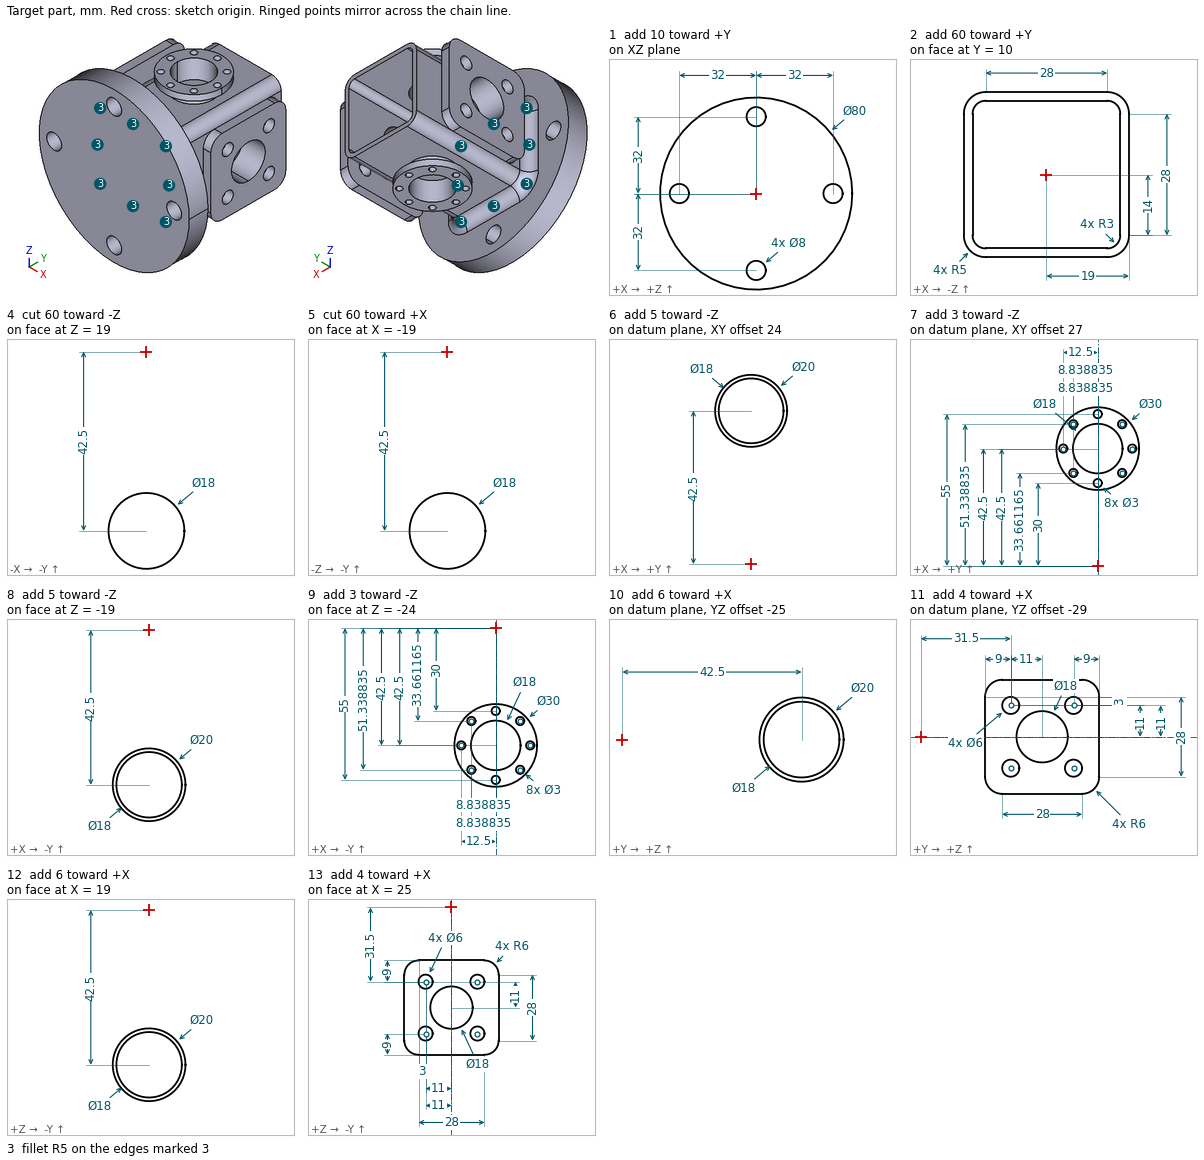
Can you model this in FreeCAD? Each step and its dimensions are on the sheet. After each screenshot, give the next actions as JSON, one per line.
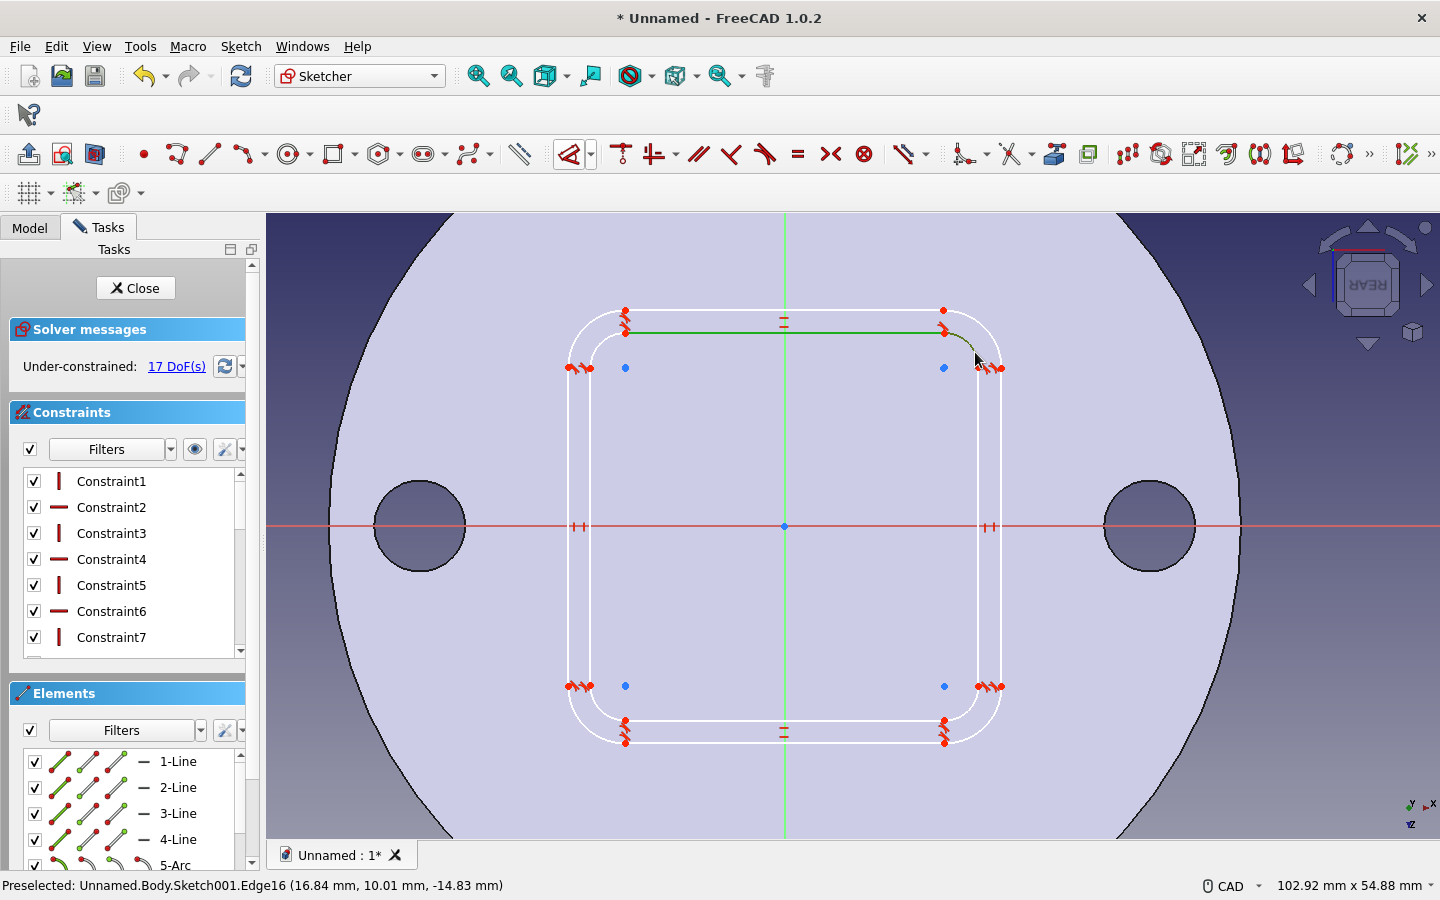
{"action": "key", "text": "t"}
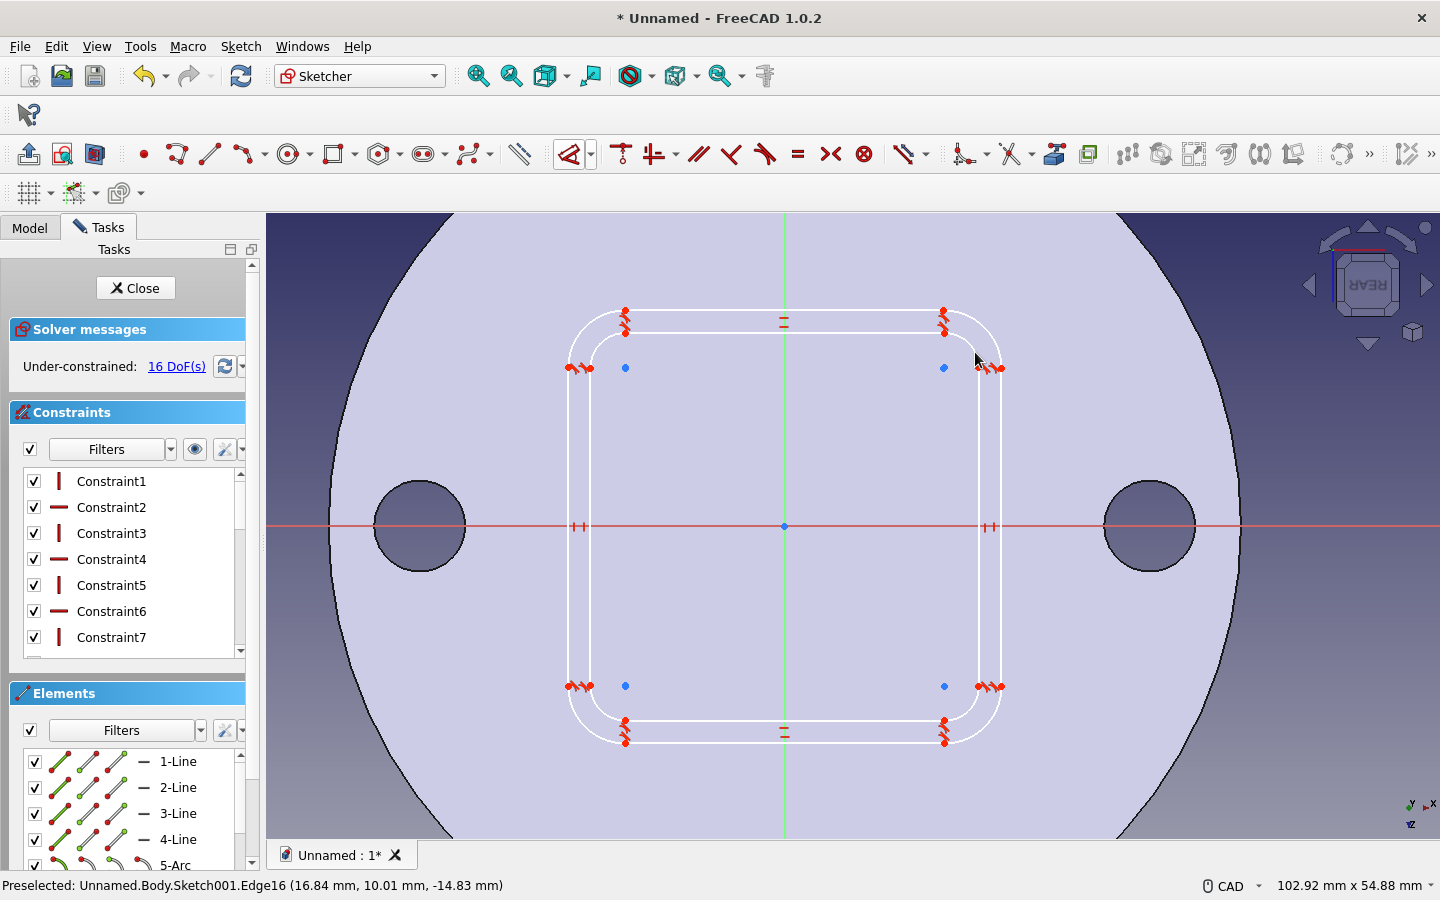
{"action": "left_click", "coordinate": [970, 737]}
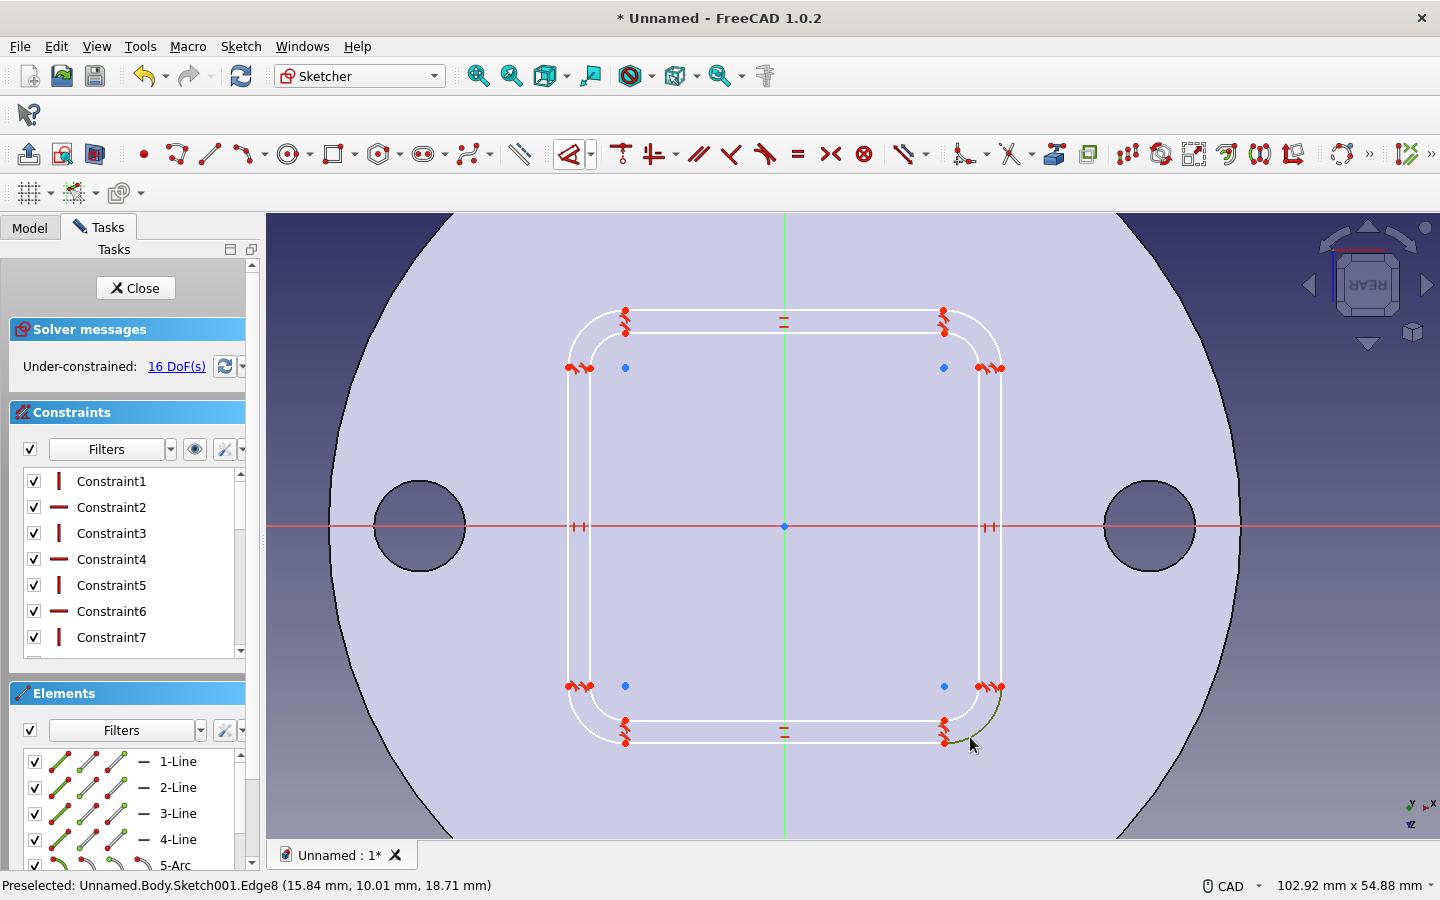
{"action": "left_click", "coordinate": [960, 717]}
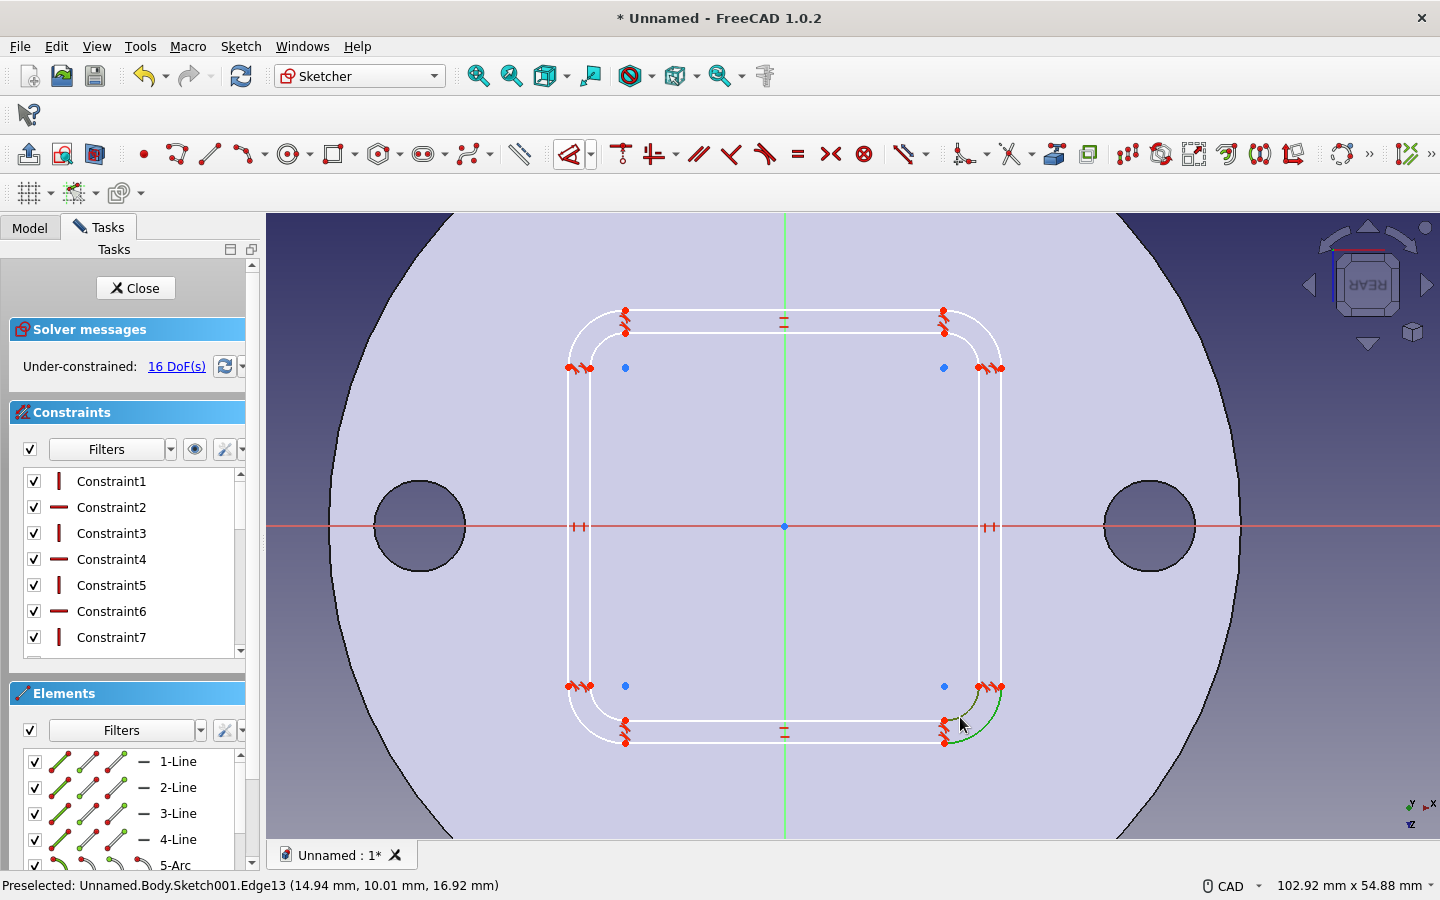
{"action": "key", "text": "c"}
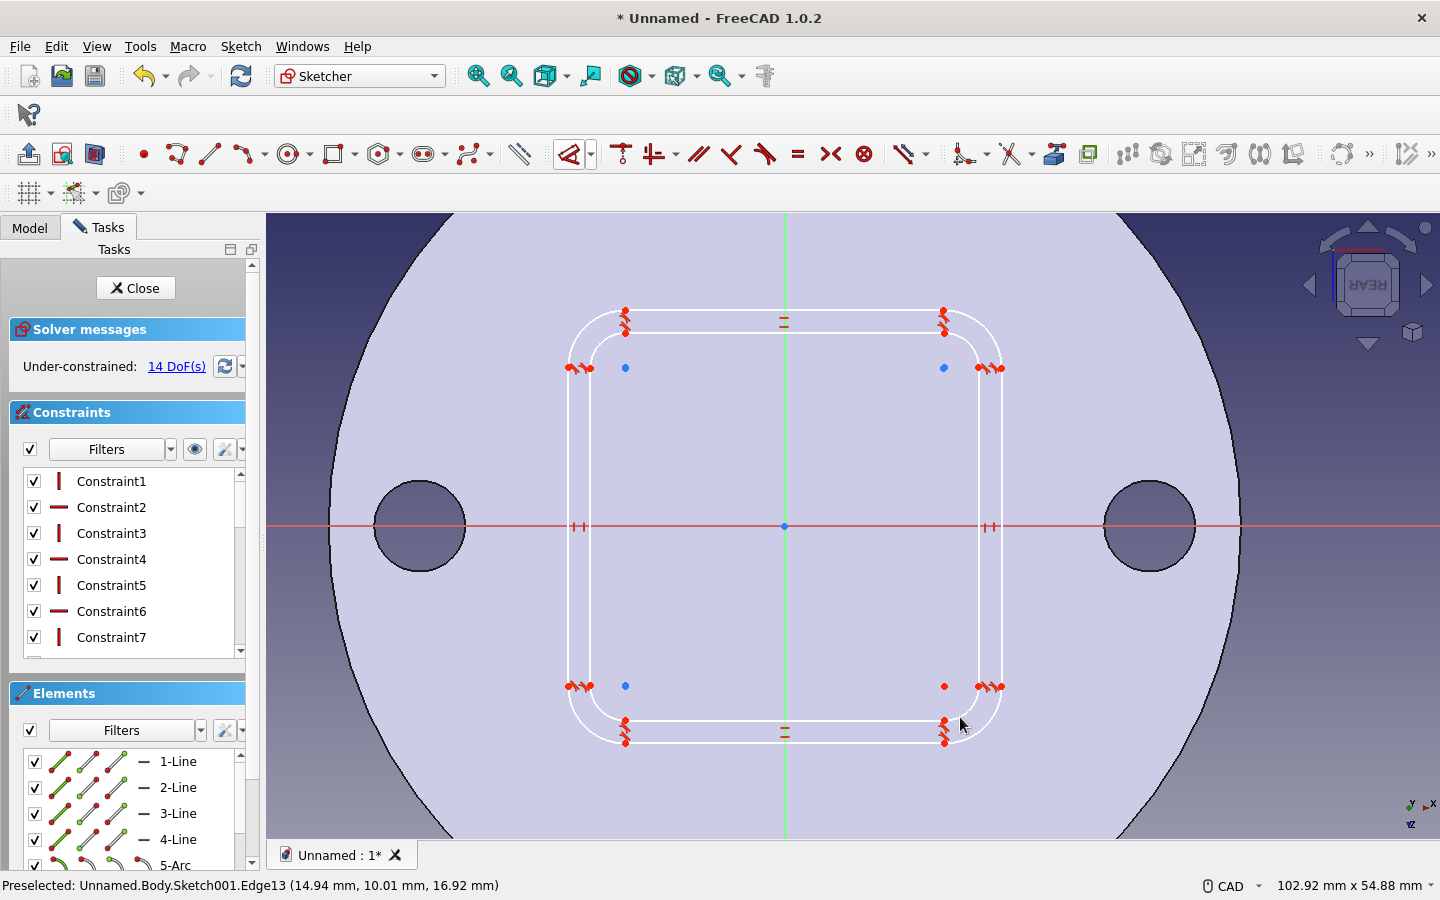
{"action": "left_click", "coordinate": [575, 712]}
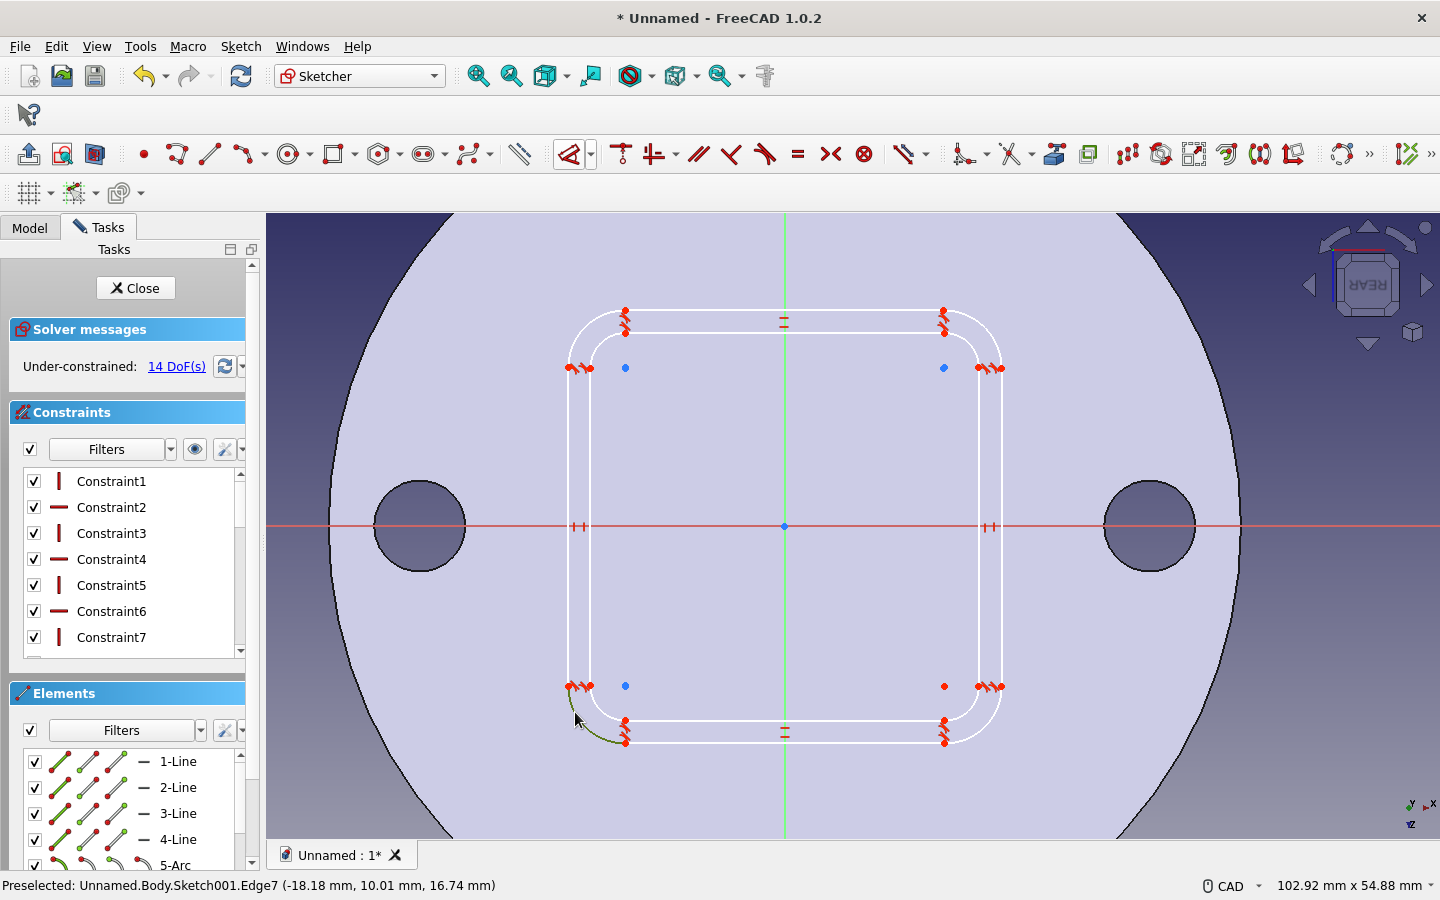
{"action": "left_click", "coordinate": [594, 701]}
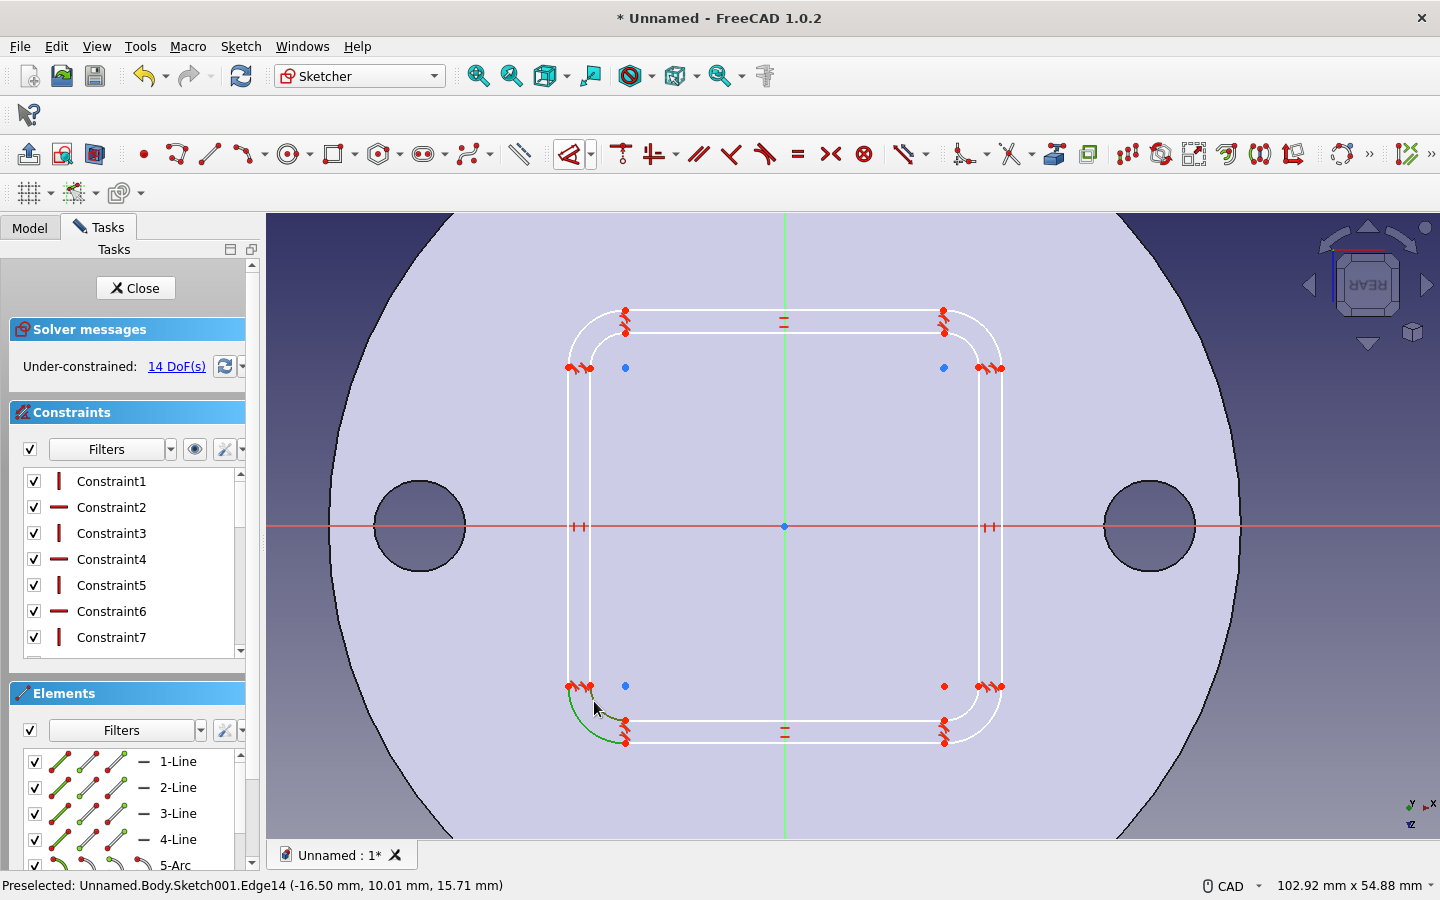
{"action": "key", "text": "c"}